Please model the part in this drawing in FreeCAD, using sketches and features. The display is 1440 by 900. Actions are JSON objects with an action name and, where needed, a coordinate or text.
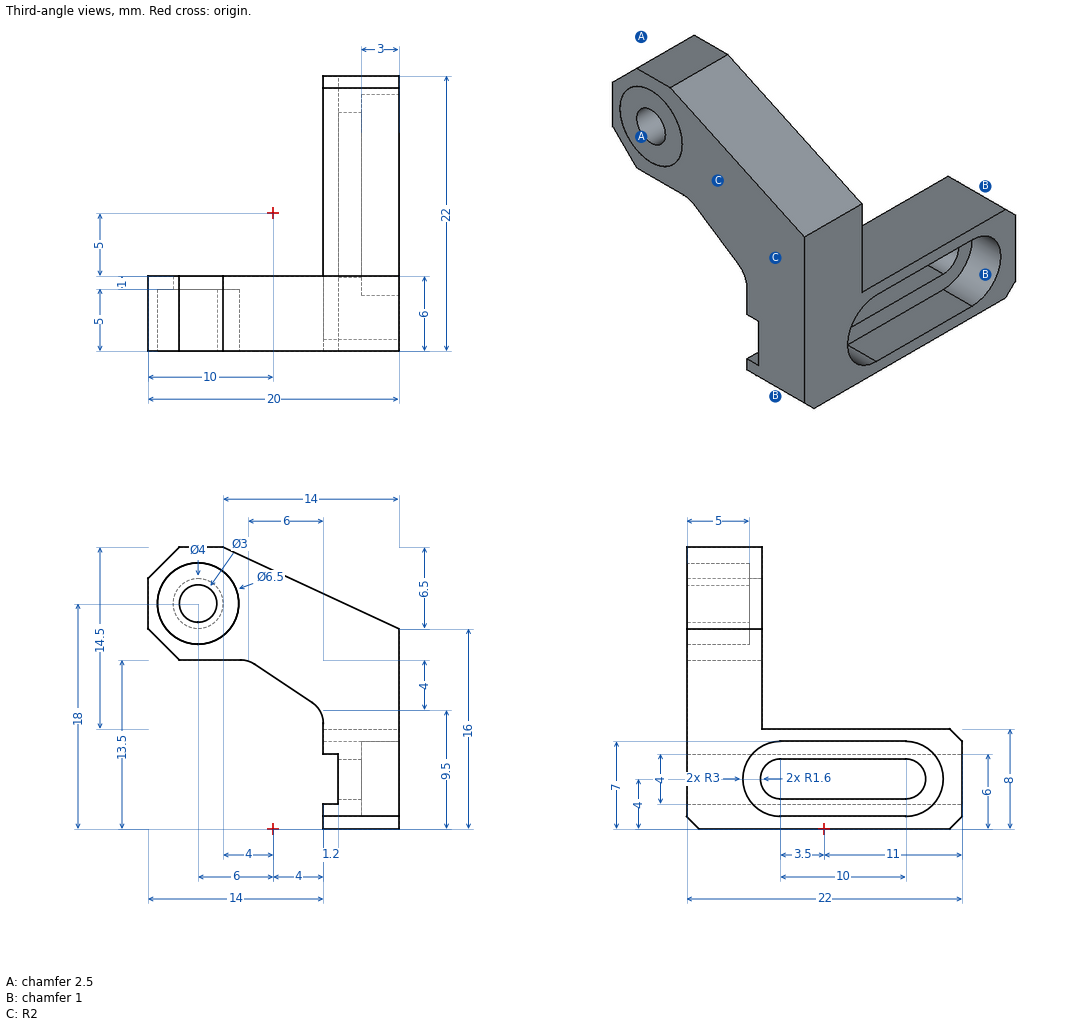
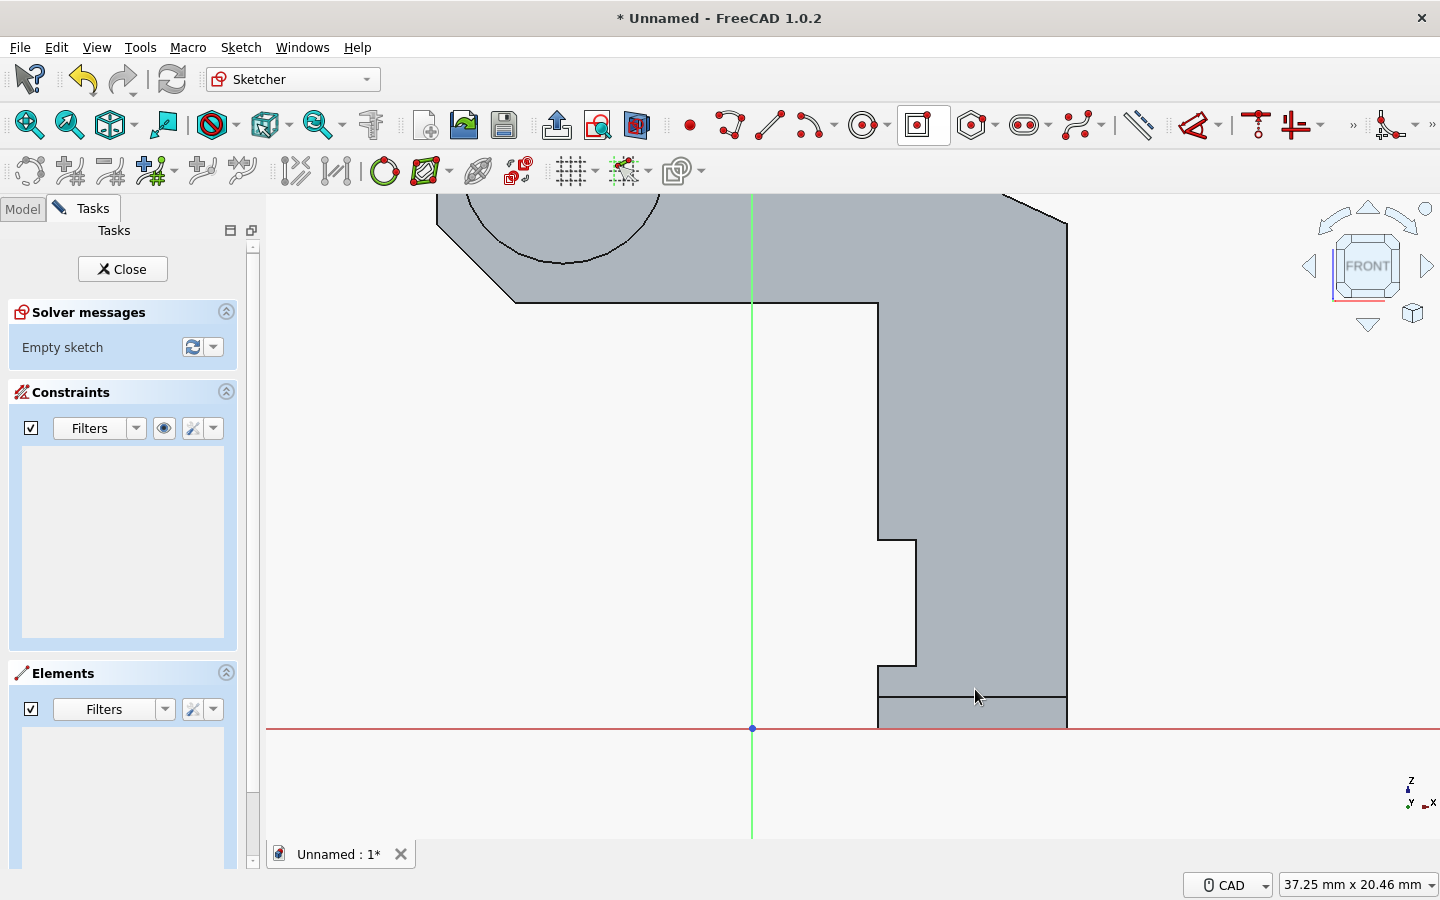
{"action": "left_click", "coordinate": [730, 126]}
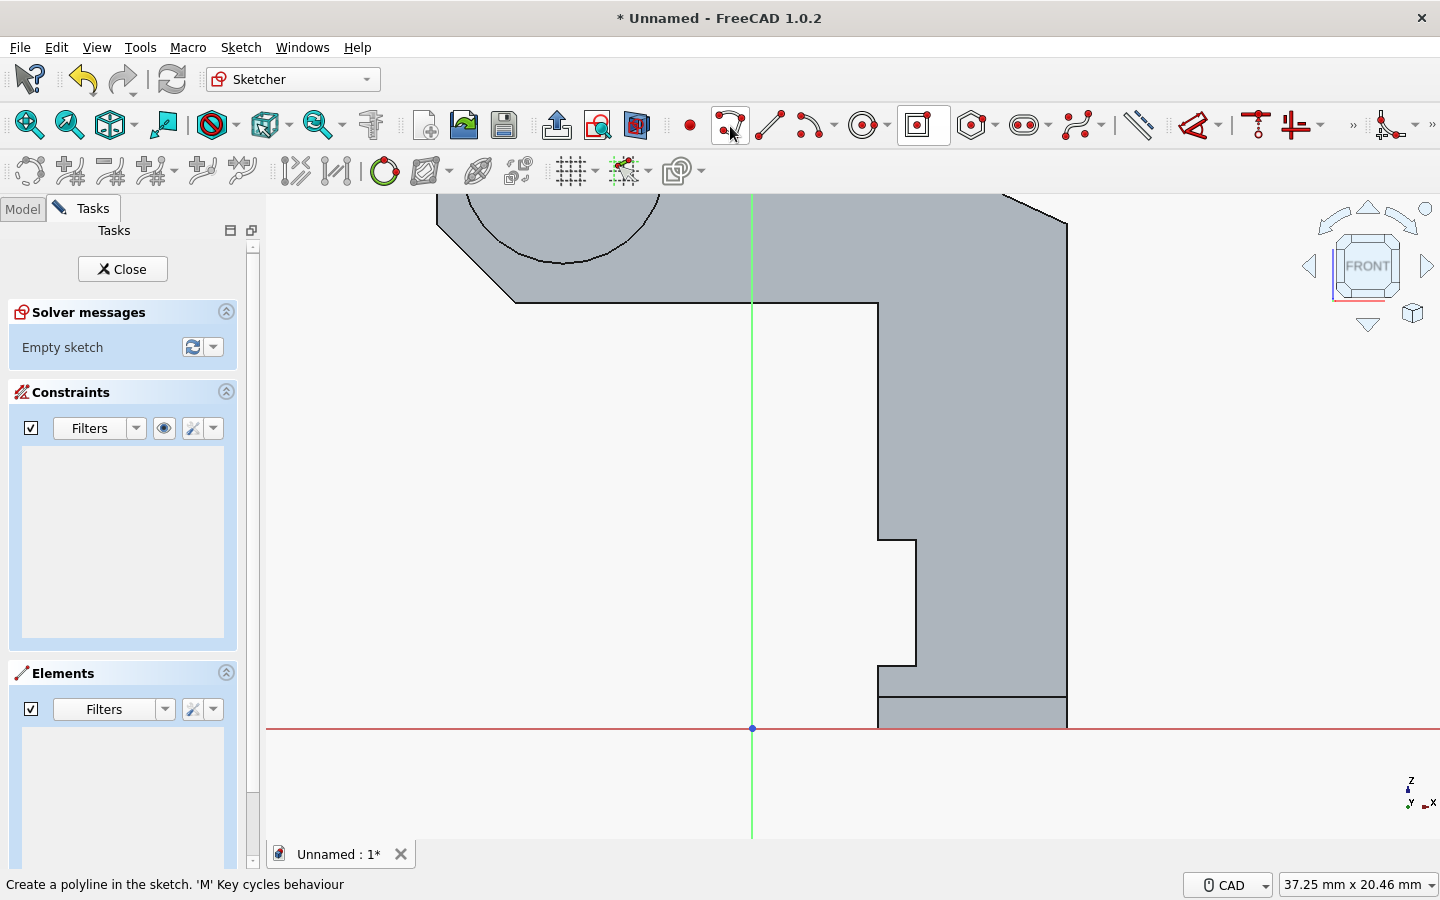
{"action": "left_click", "coordinate": [878, 429]}
{"action": "left_click", "coordinate": [878, 303]}
{"action": "left_click", "coordinate": [689, 303]}
{"action": "left_click", "coordinate": [878, 430]}
{"action": "key", "text": "Escape"}
{"action": "key", "text": "Escape"}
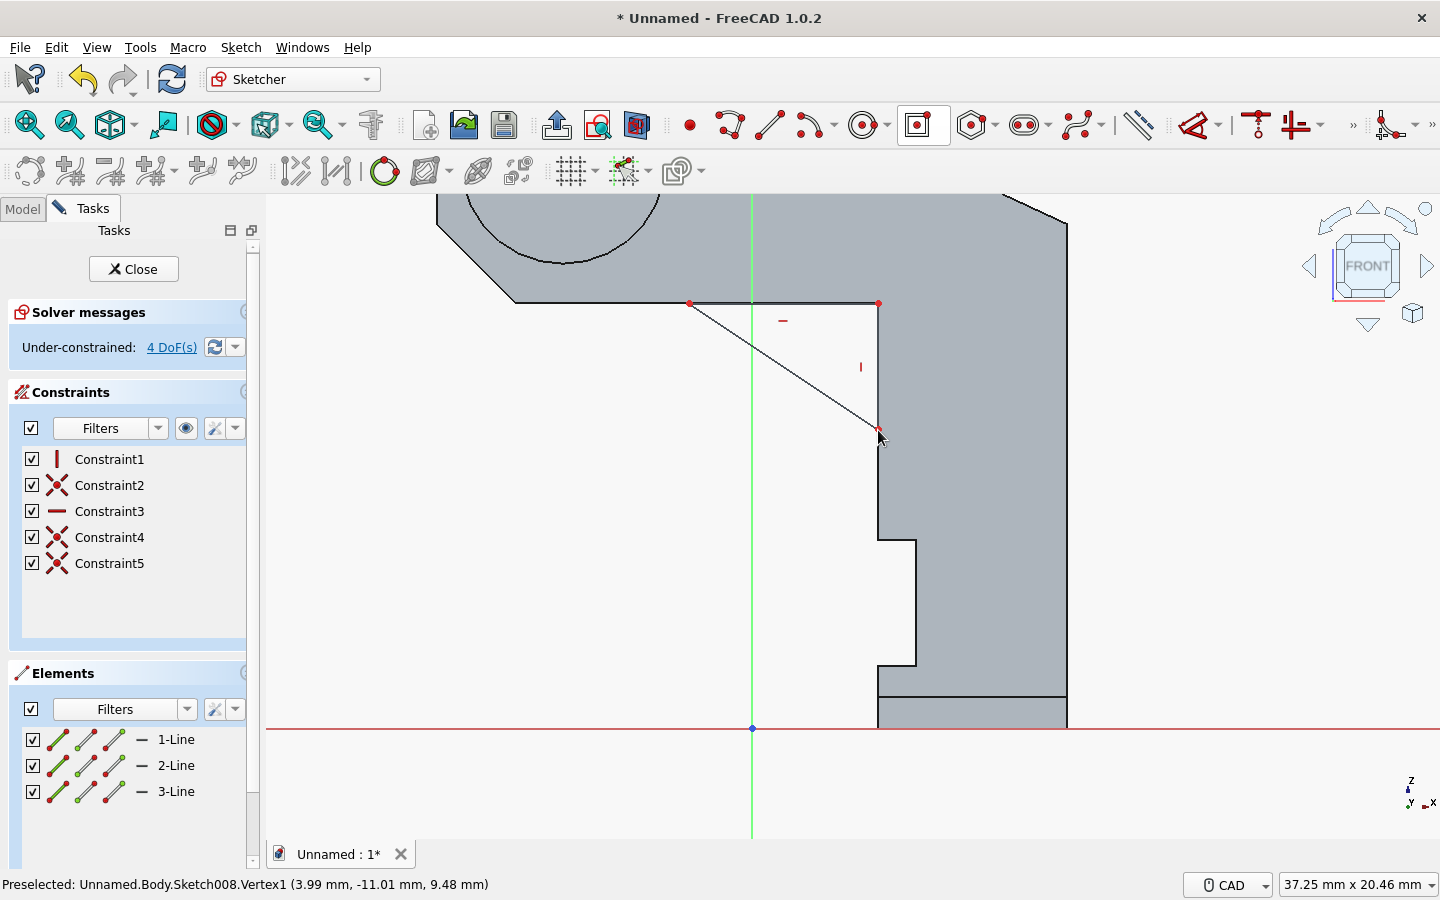
{"action": "left_click", "coordinate": [1194, 126]}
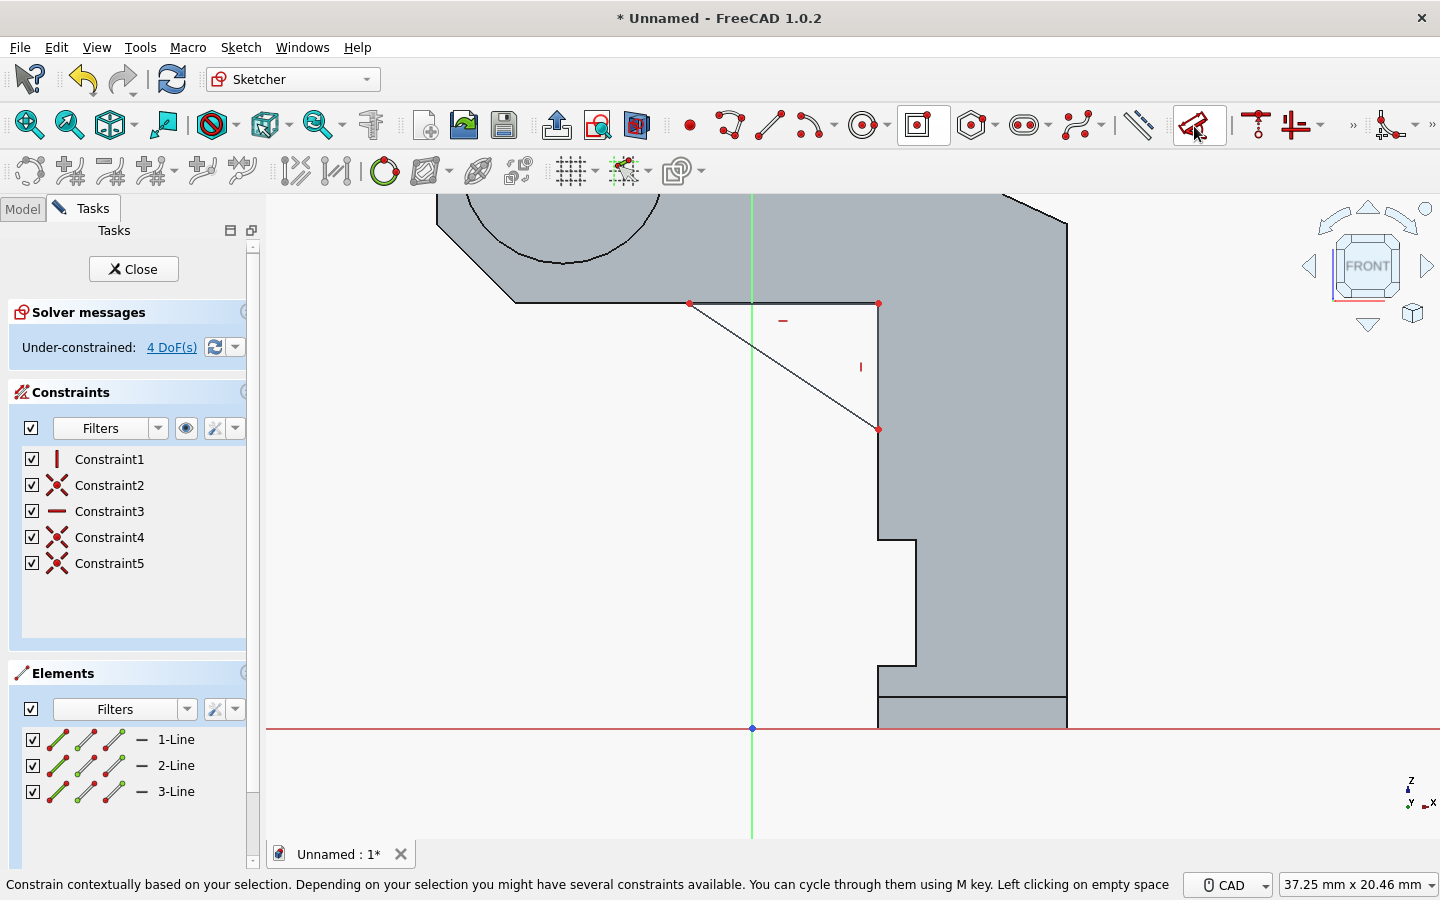
{"action": "left_click", "coordinate": [878, 392]}
{"action": "left_click", "coordinate": [912, 367]}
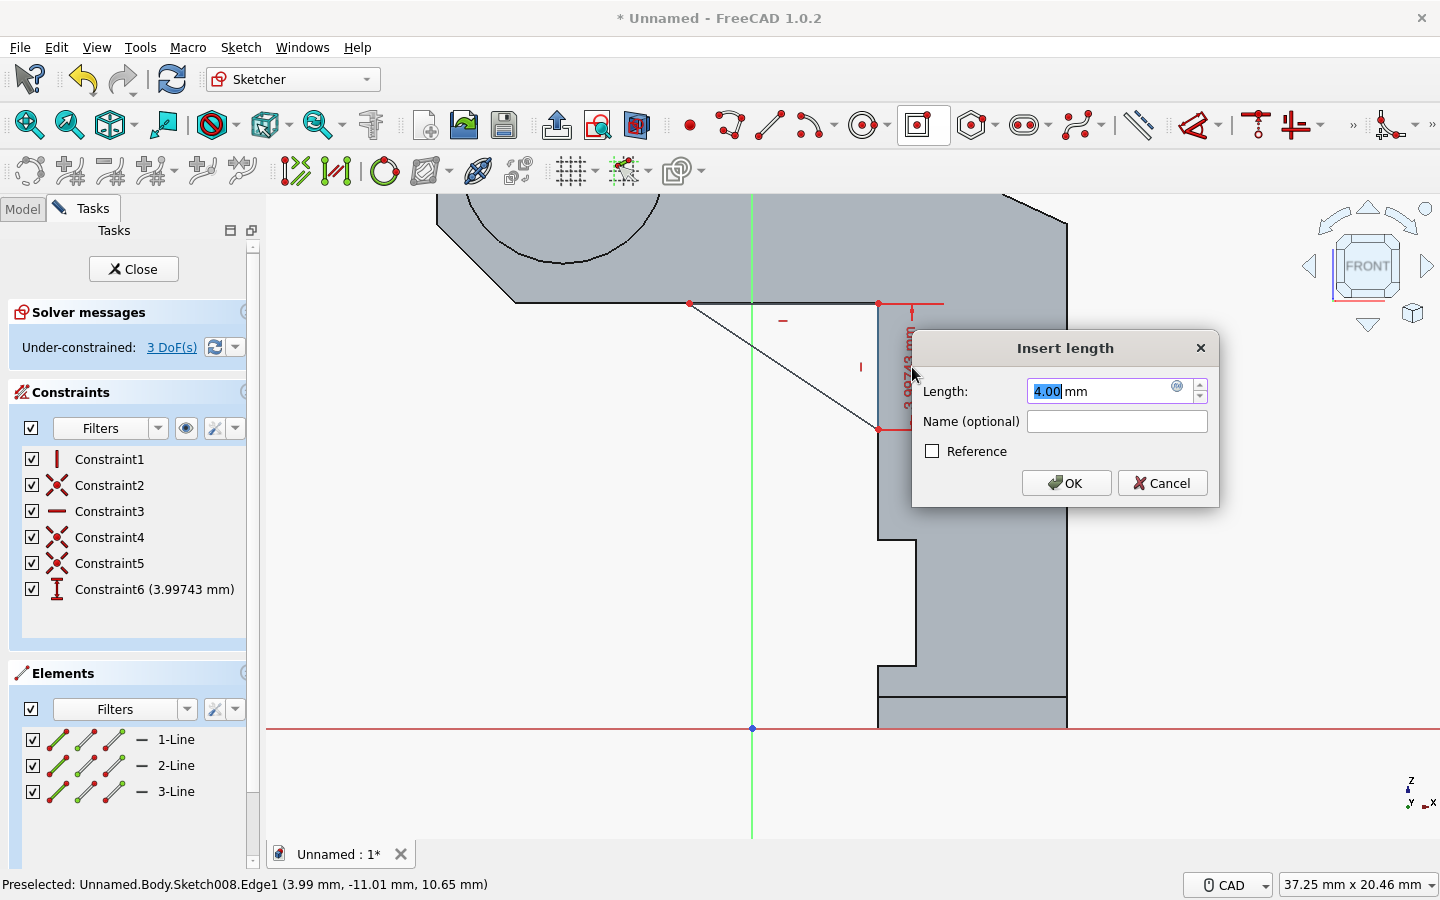
{"action": "type", "text": "4"}
{"action": "key", "text": "Return"}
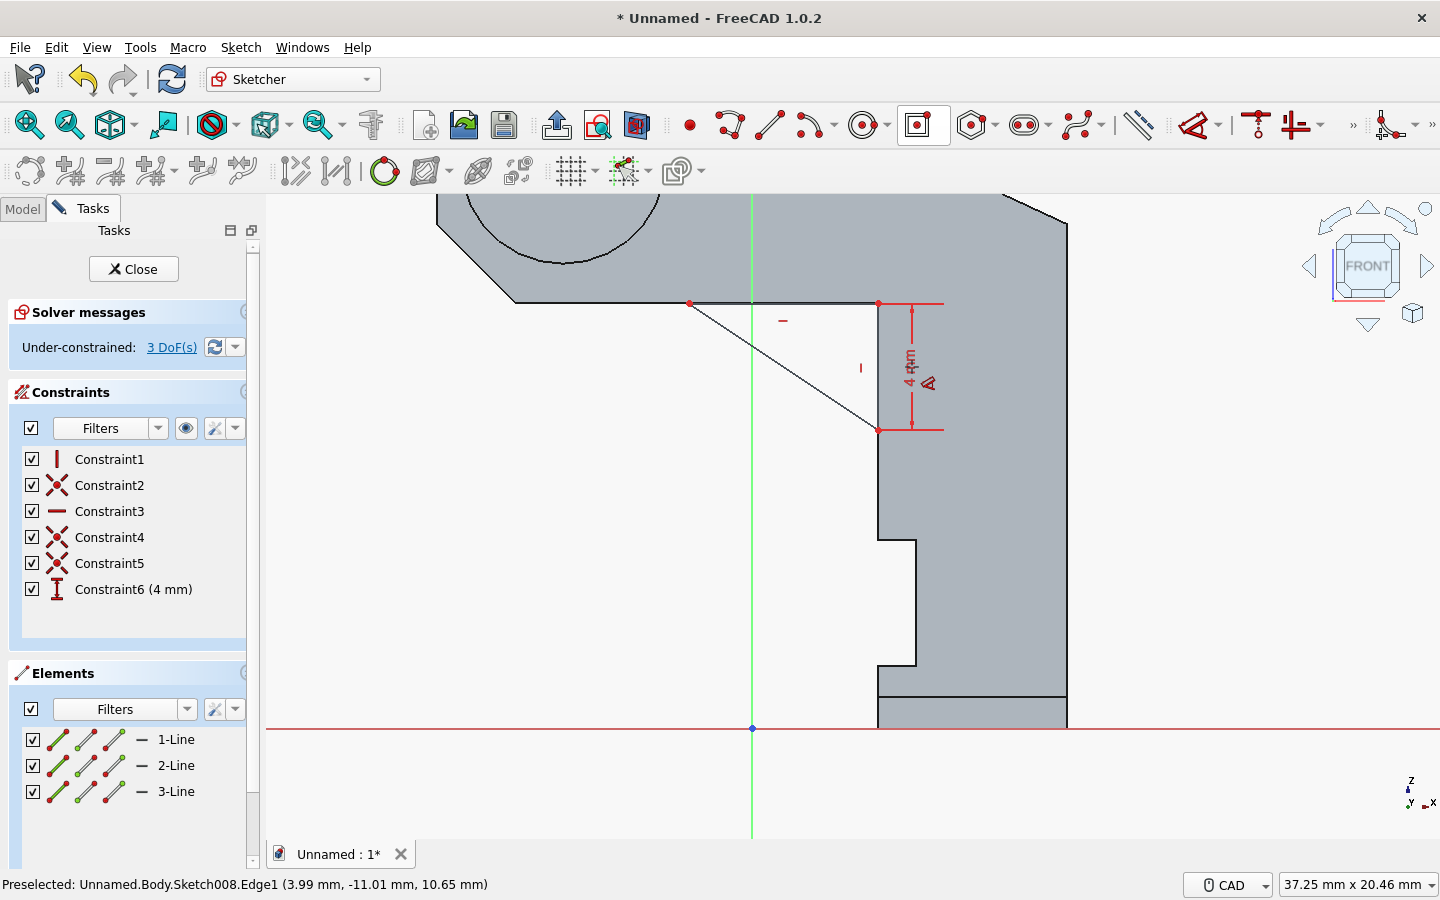
{"action": "left_click", "coordinate": [821, 304]}
{"action": "left_click", "coordinate": [784, 270]}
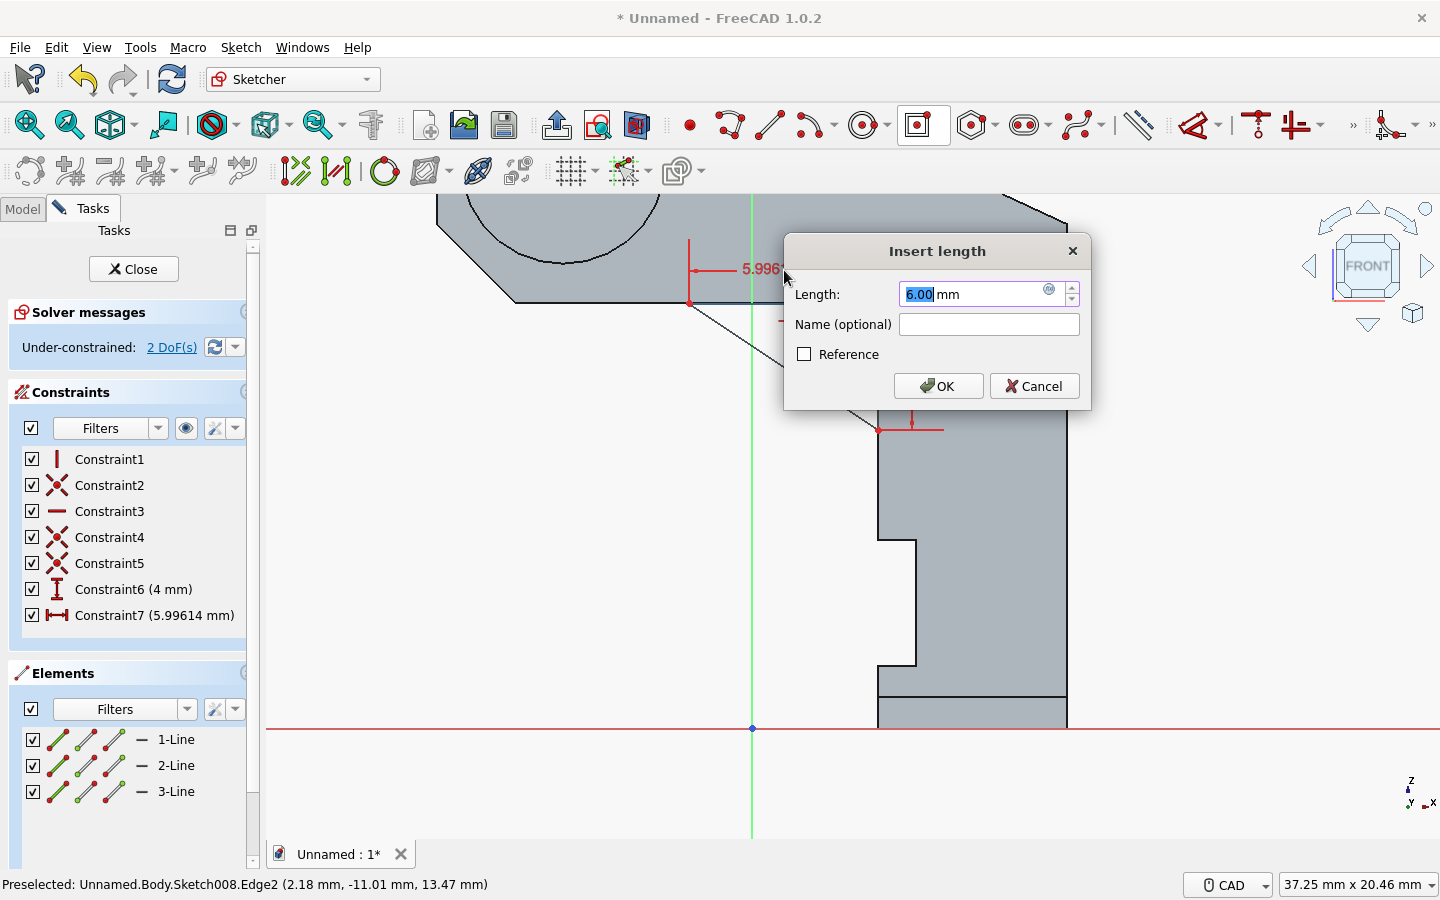
{"action": "type", "text": "6"}
{"action": "key", "text": "Return"}